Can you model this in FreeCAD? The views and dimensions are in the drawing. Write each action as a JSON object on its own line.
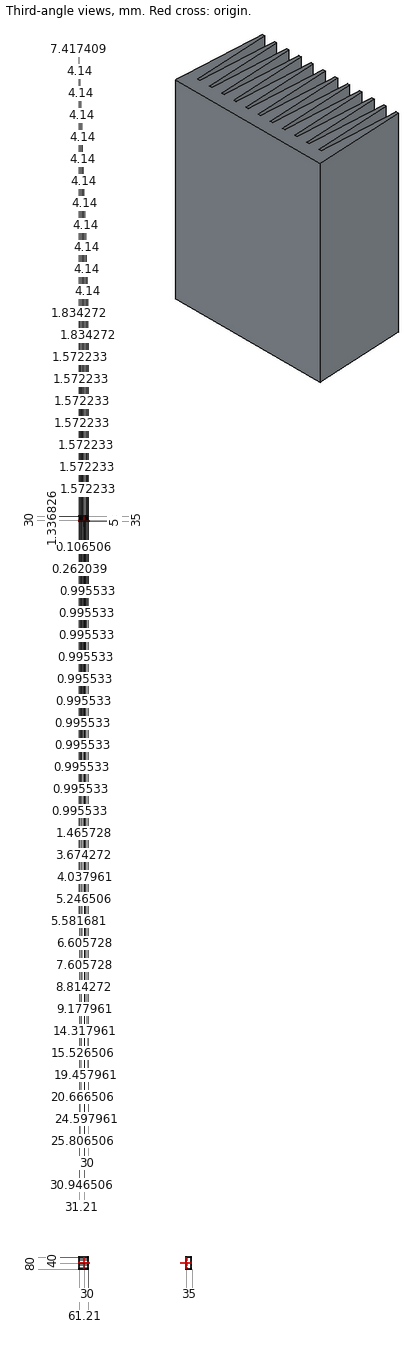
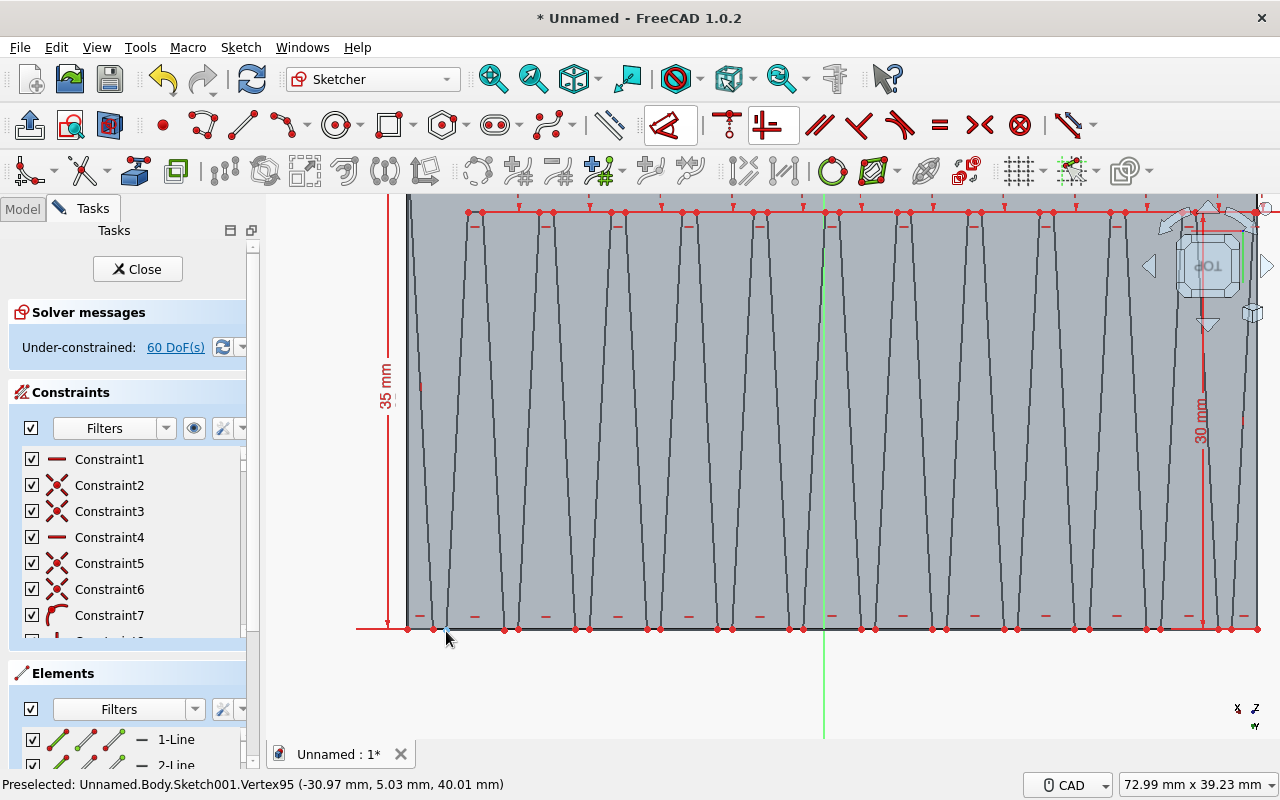
{"action": "left_click", "coordinate": [446, 630]}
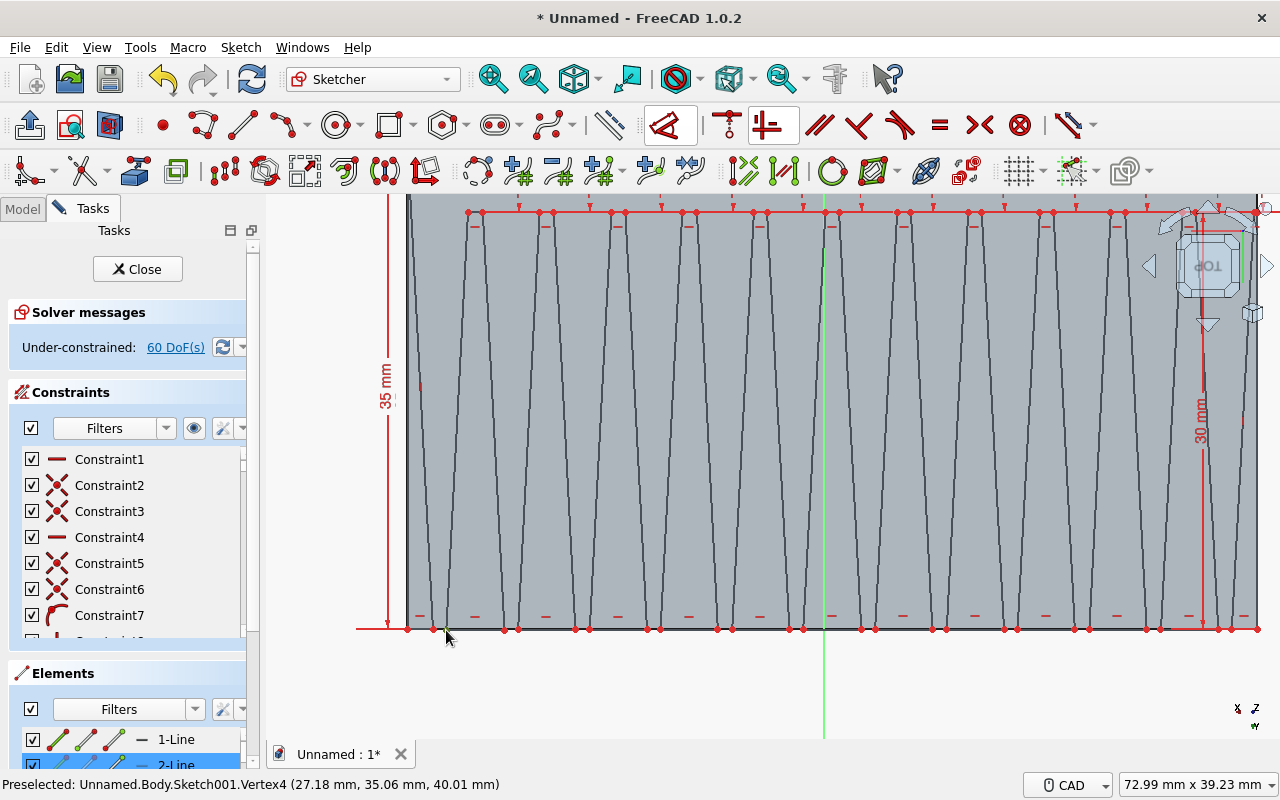
{"action": "key", "text": "i"}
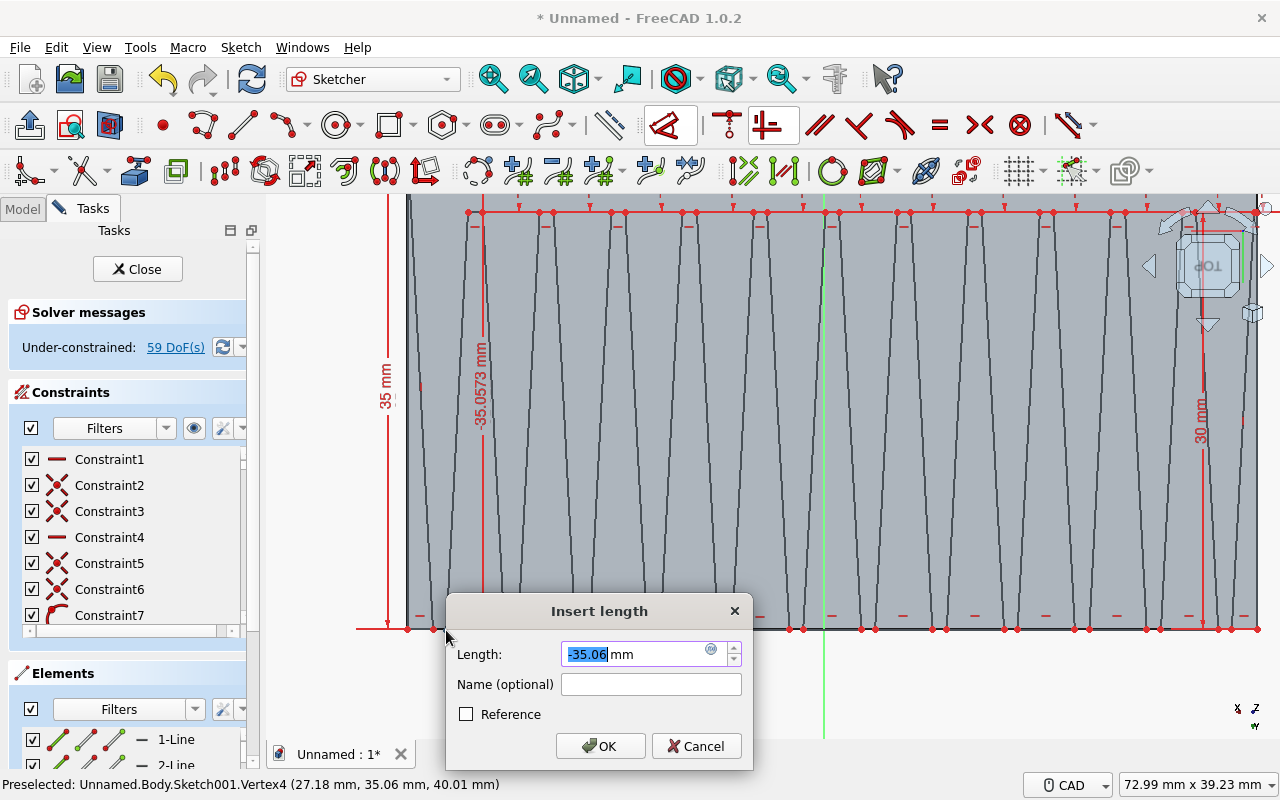
{"action": "type", "text": "-35"}
{"action": "key", "text": "Return"}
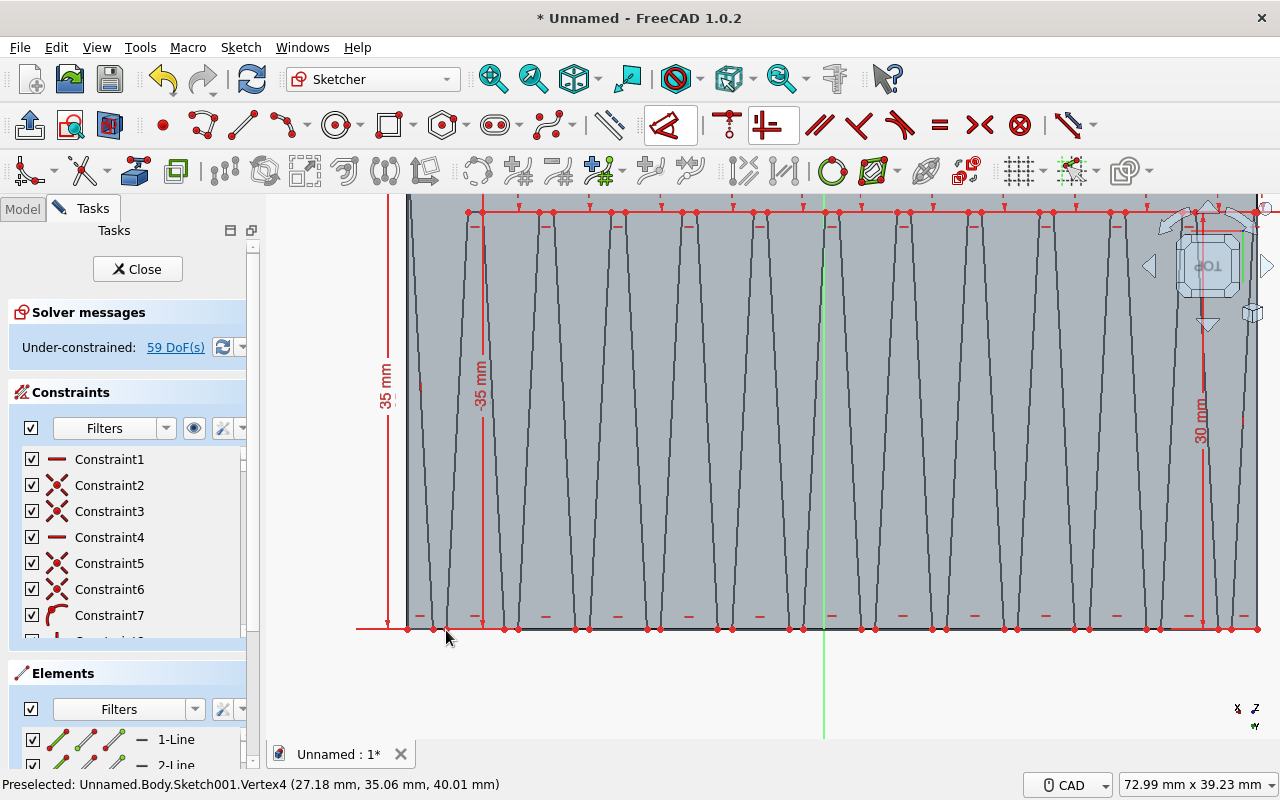
{"action": "scroll", "coordinate": [445, 630], "scroll_direction": "down", "scroll_amount": 2}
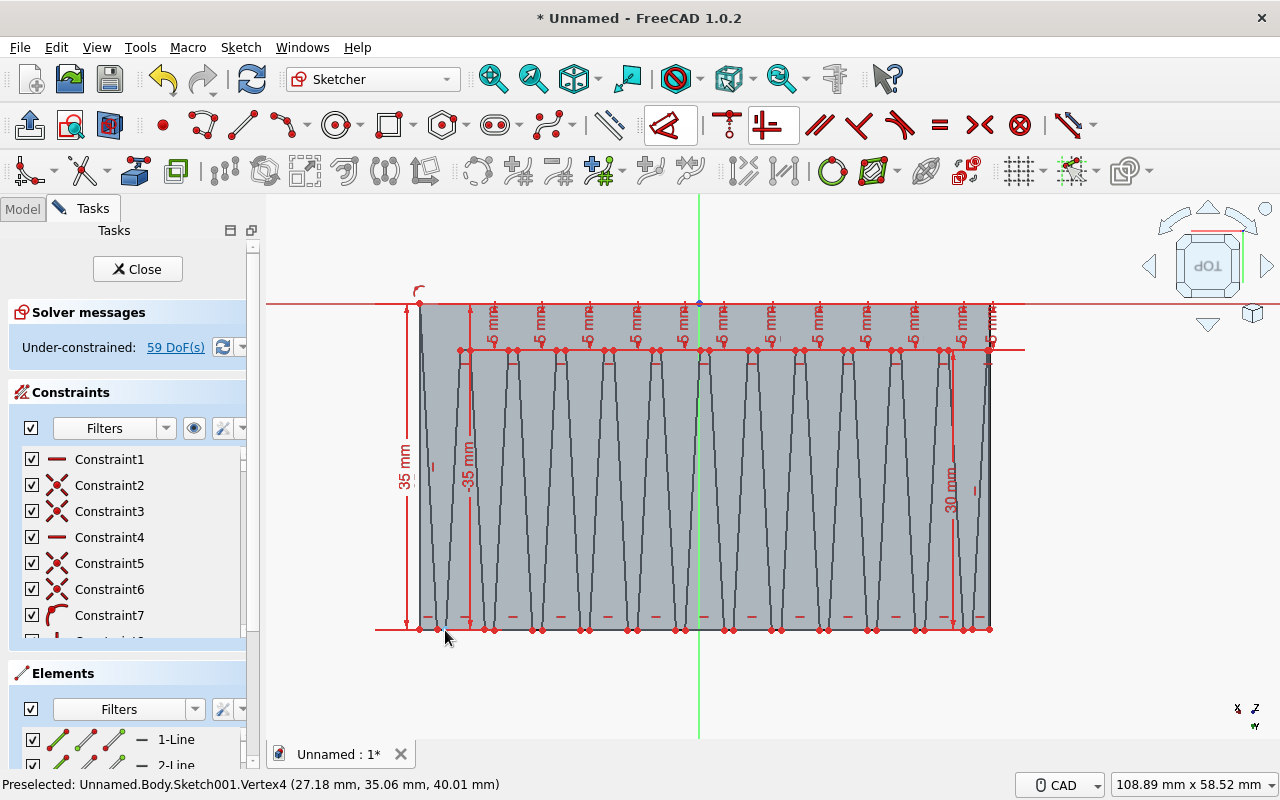
{"action": "left_click", "coordinate": [420, 304]}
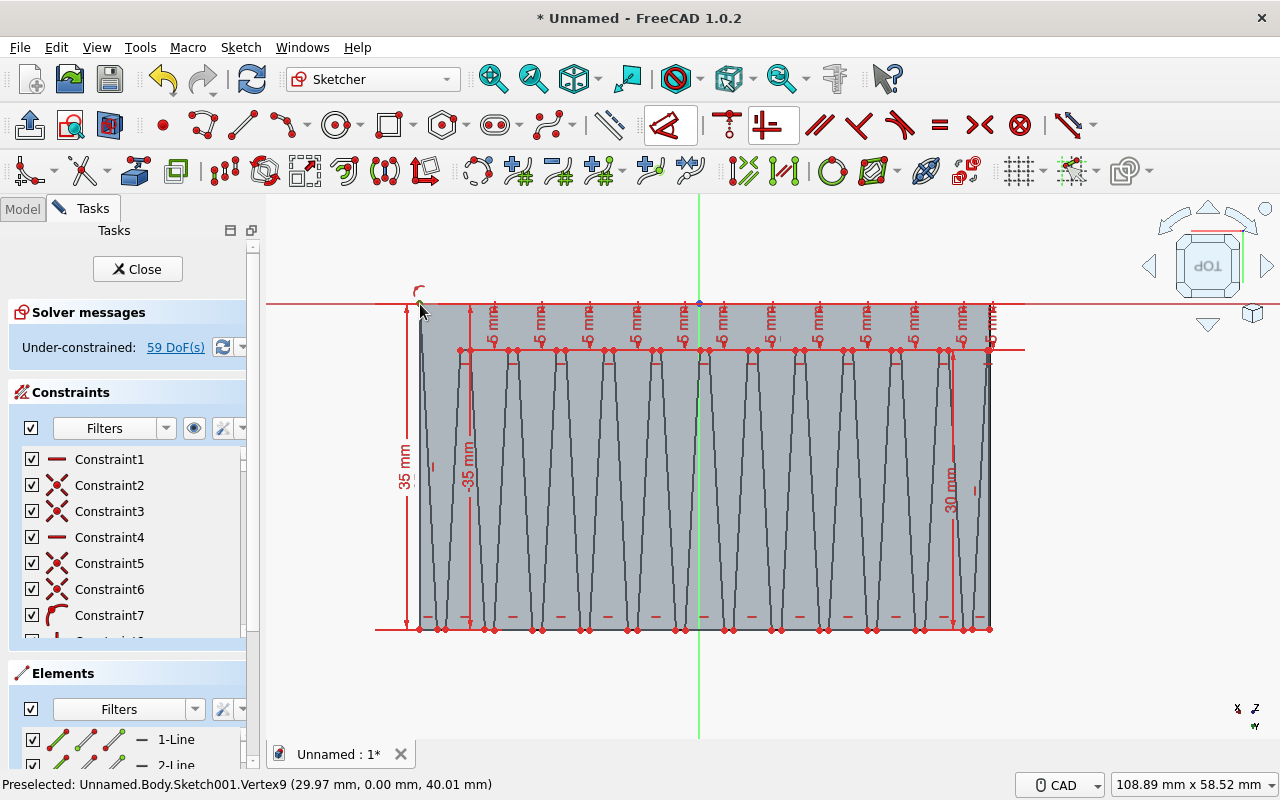
{"action": "key", "text": "l"}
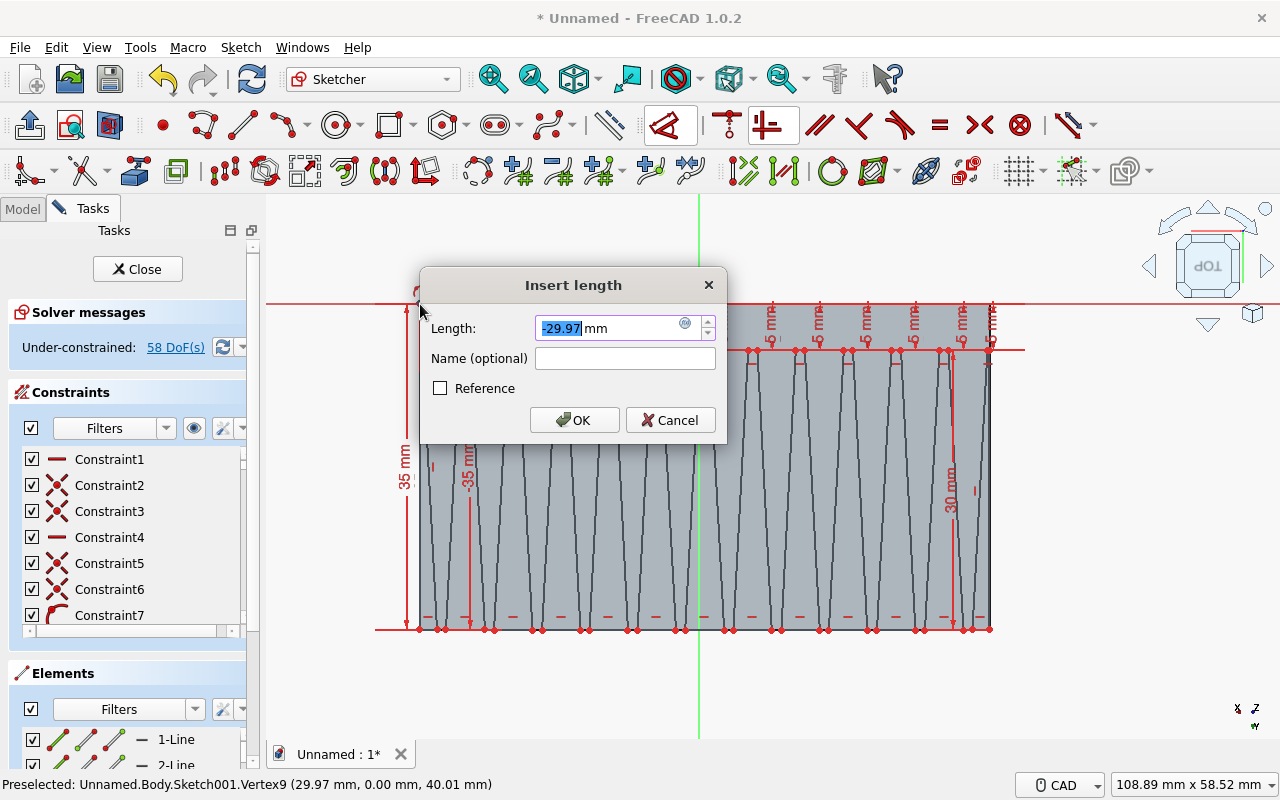
{"action": "type", "text": "-30"}
{"action": "key", "text": "Return"}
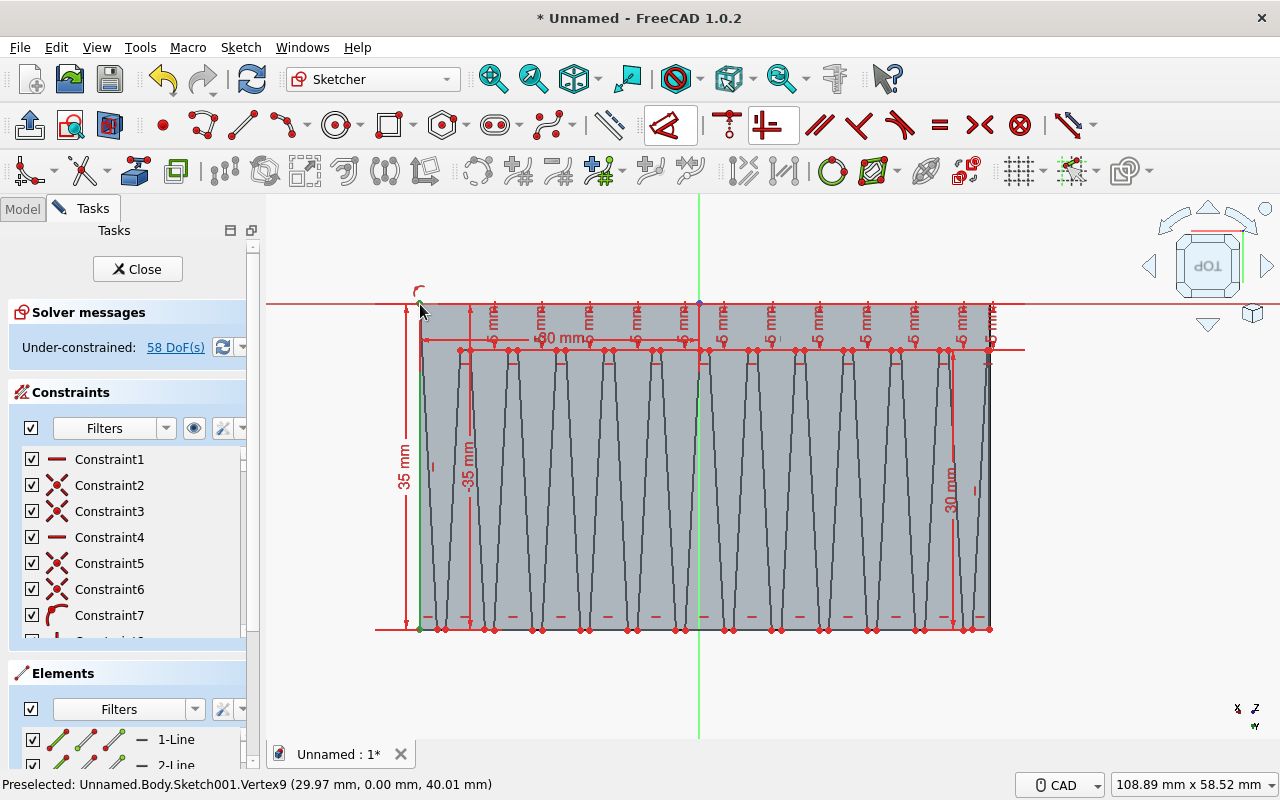
{"action": "scroll", "coordinate": [494, 630], "scroll_direction": "up", "scroll_amount": 2}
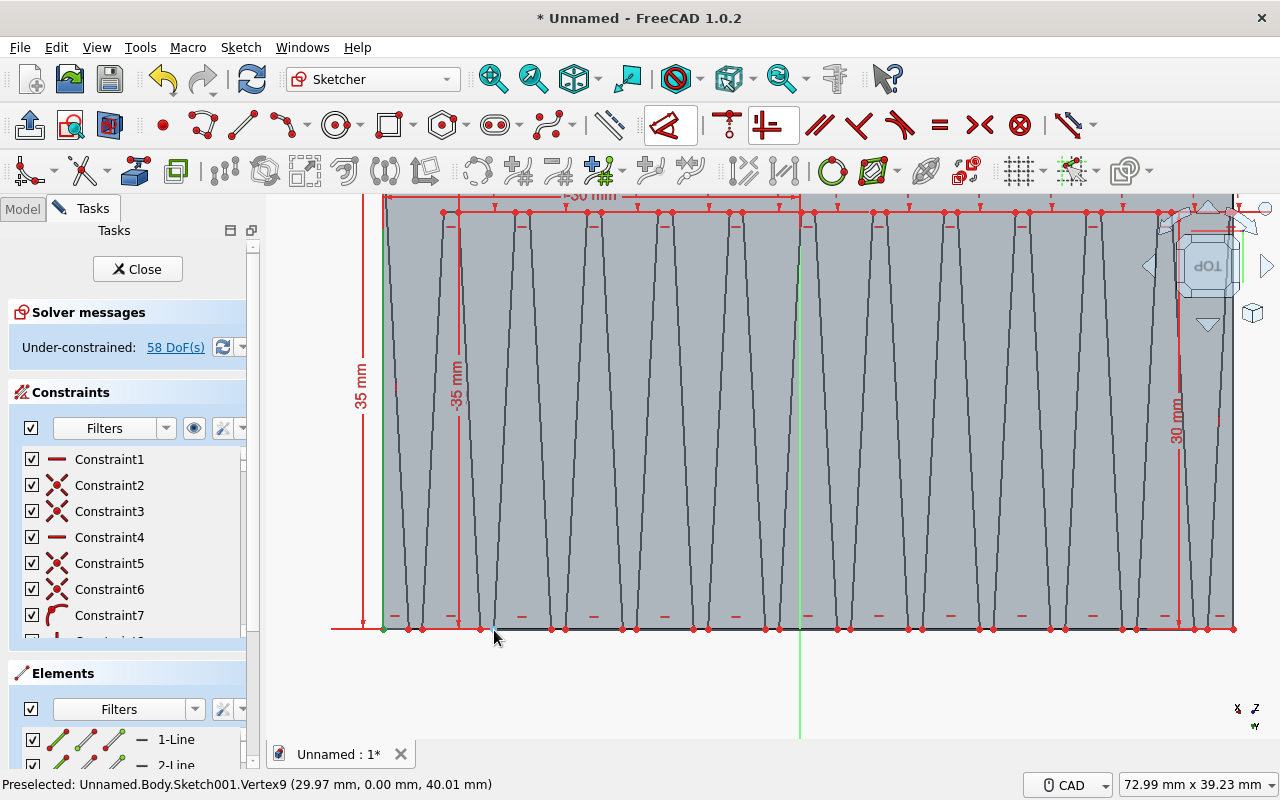
{"action": "left_click", "coordinate": [494, 630]}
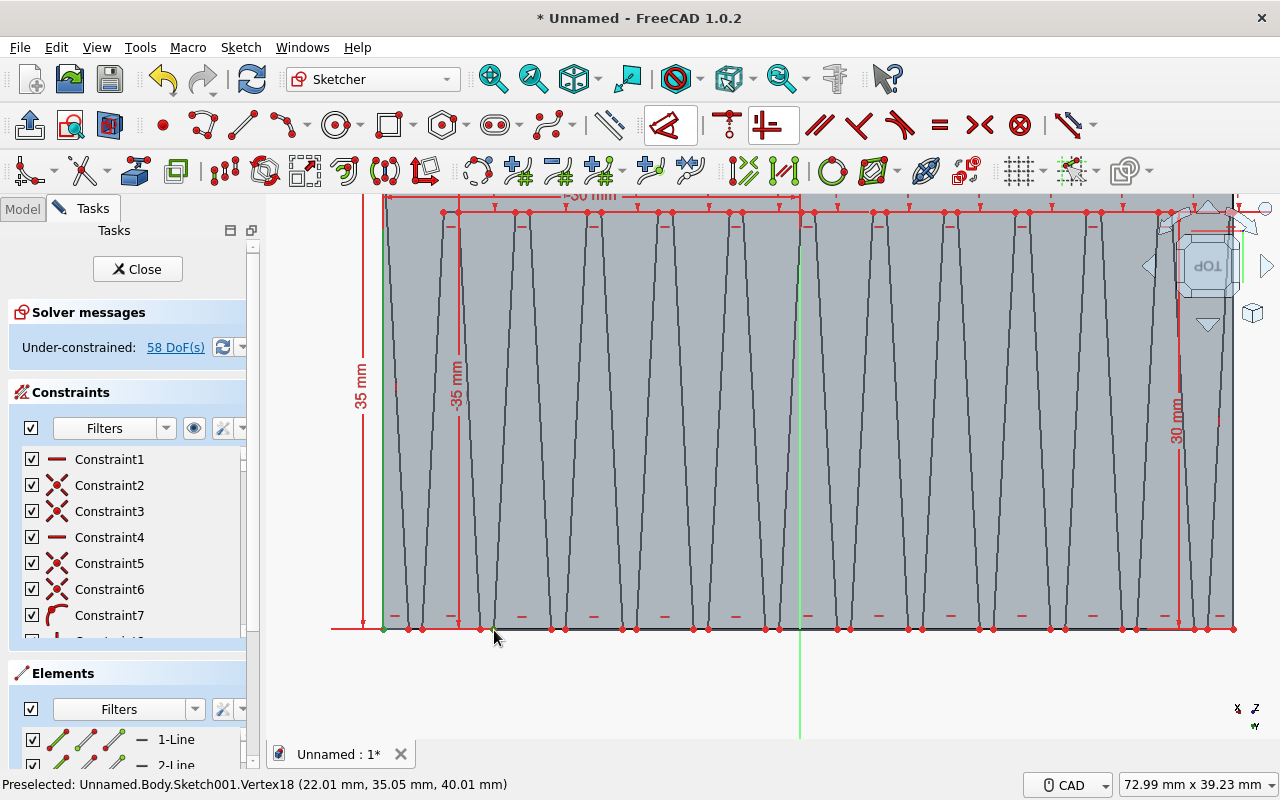
{"action": "left_click", "coordinate": [692, 126]}